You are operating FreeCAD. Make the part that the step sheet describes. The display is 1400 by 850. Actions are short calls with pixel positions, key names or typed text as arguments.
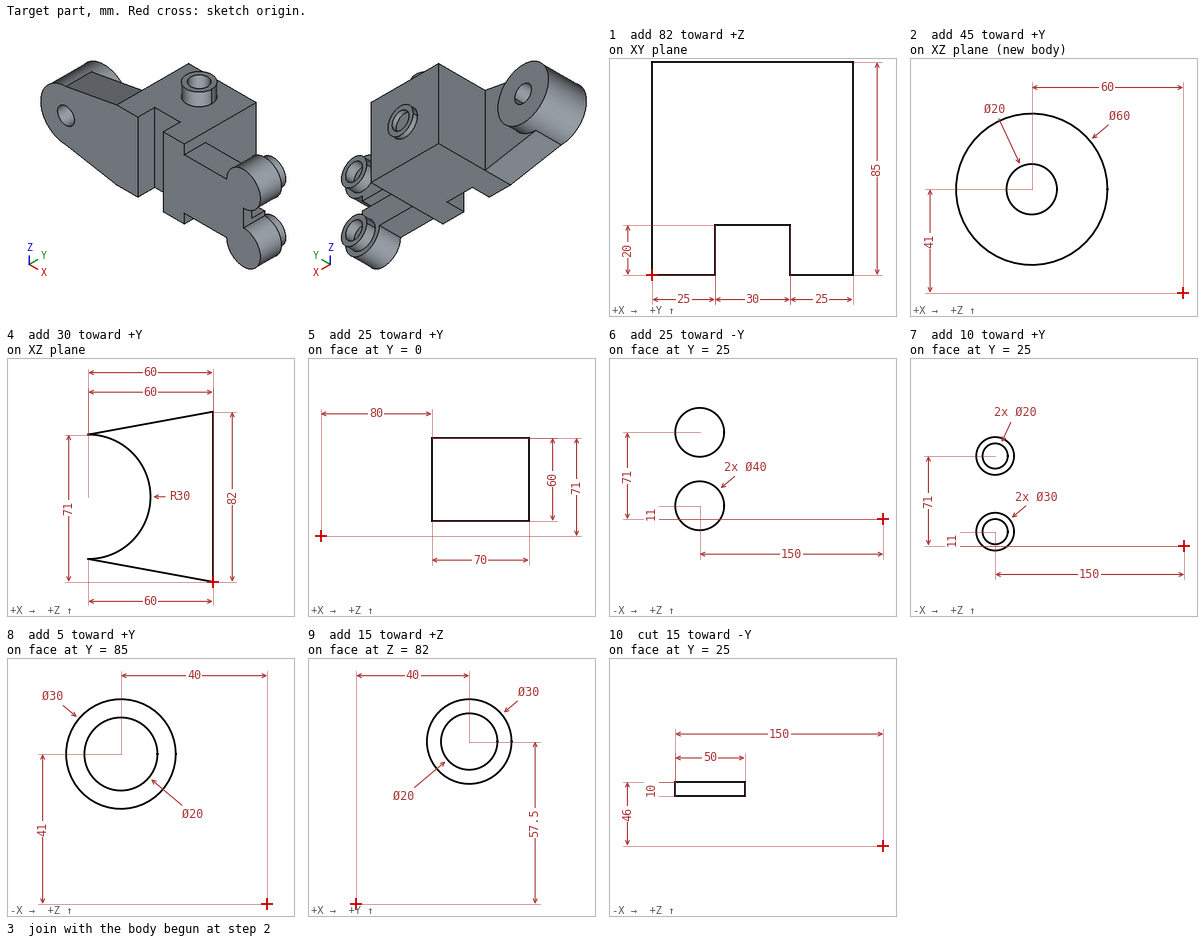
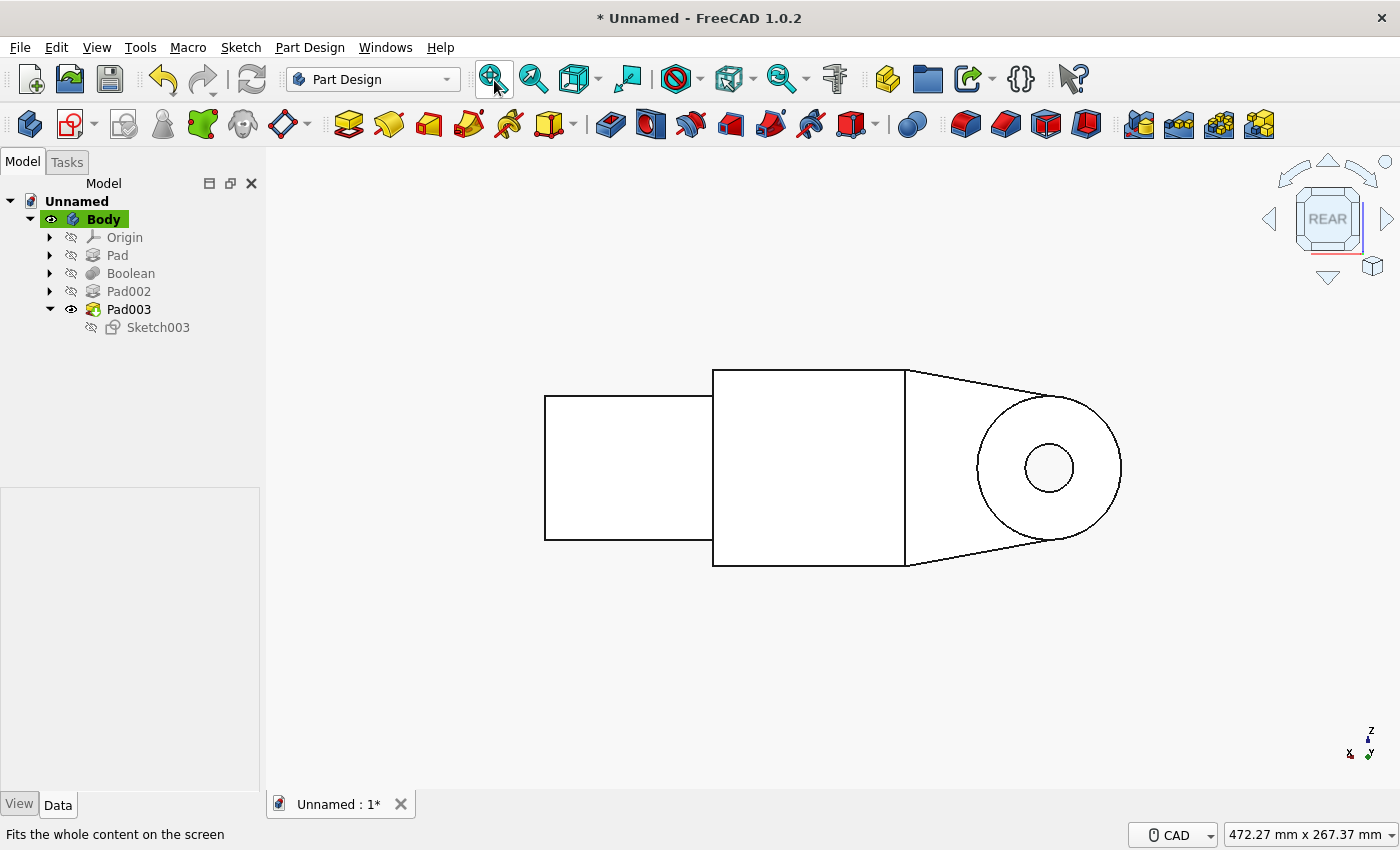
click(629, 467)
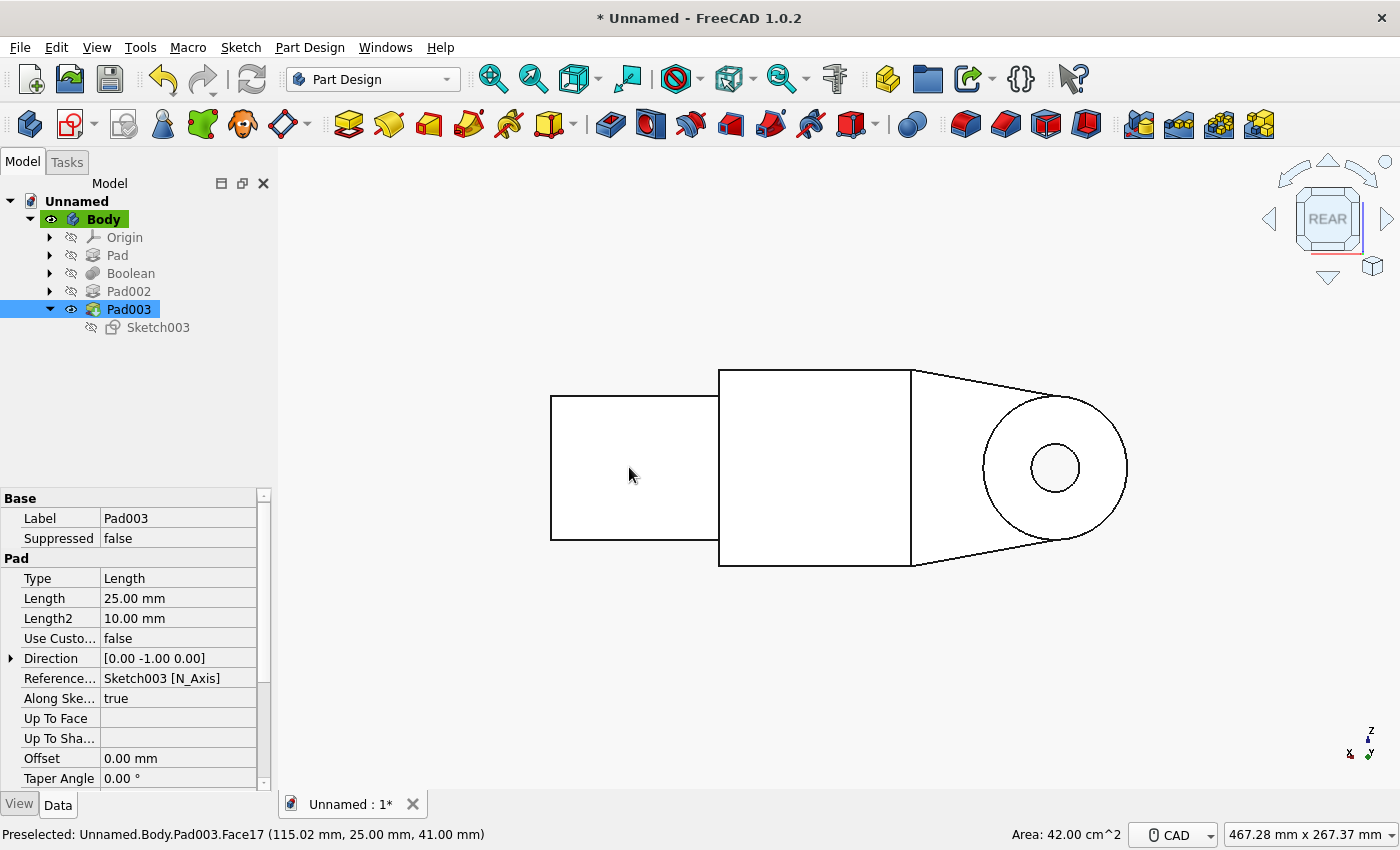
click(70, 124)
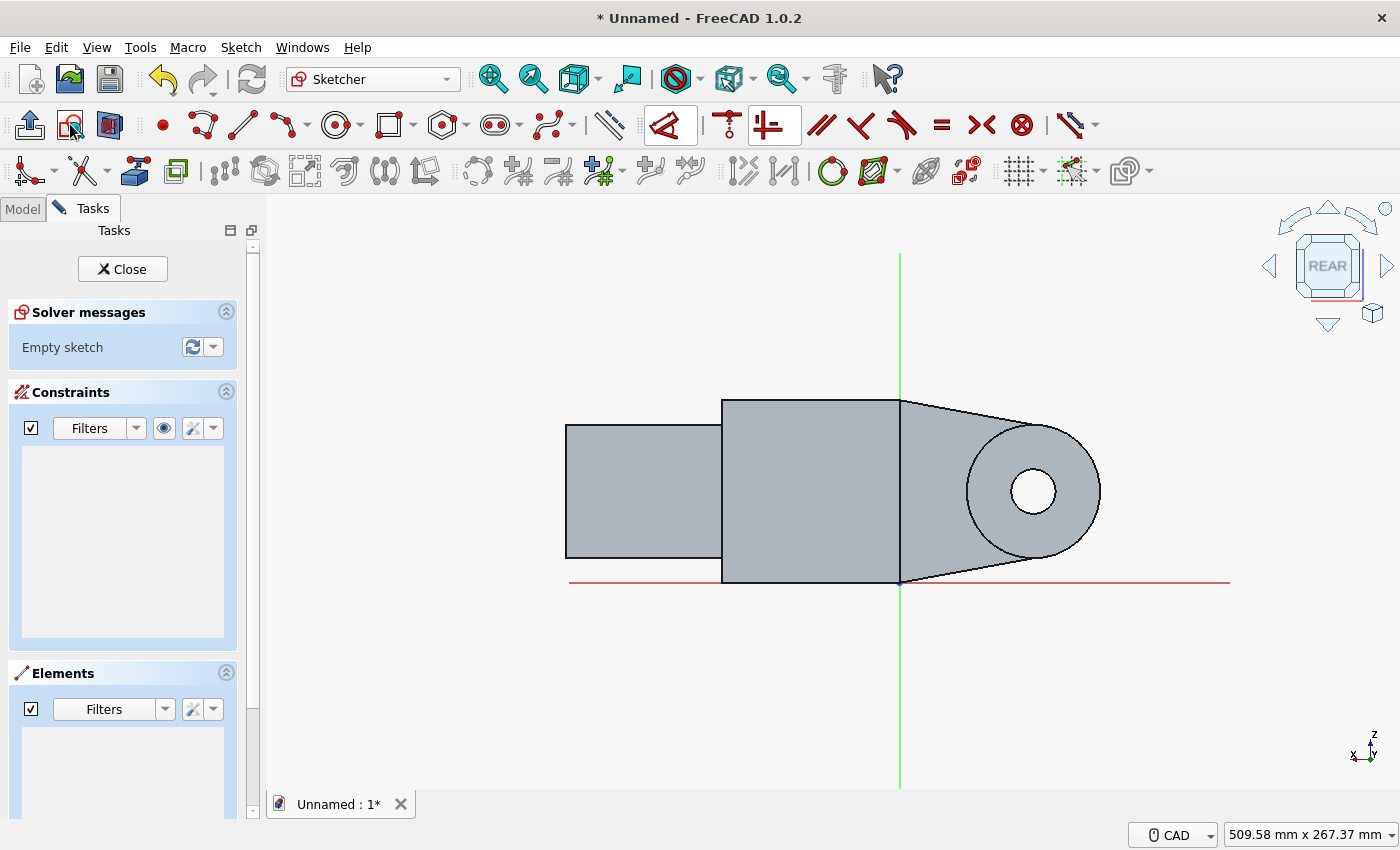
key(q)
key(s)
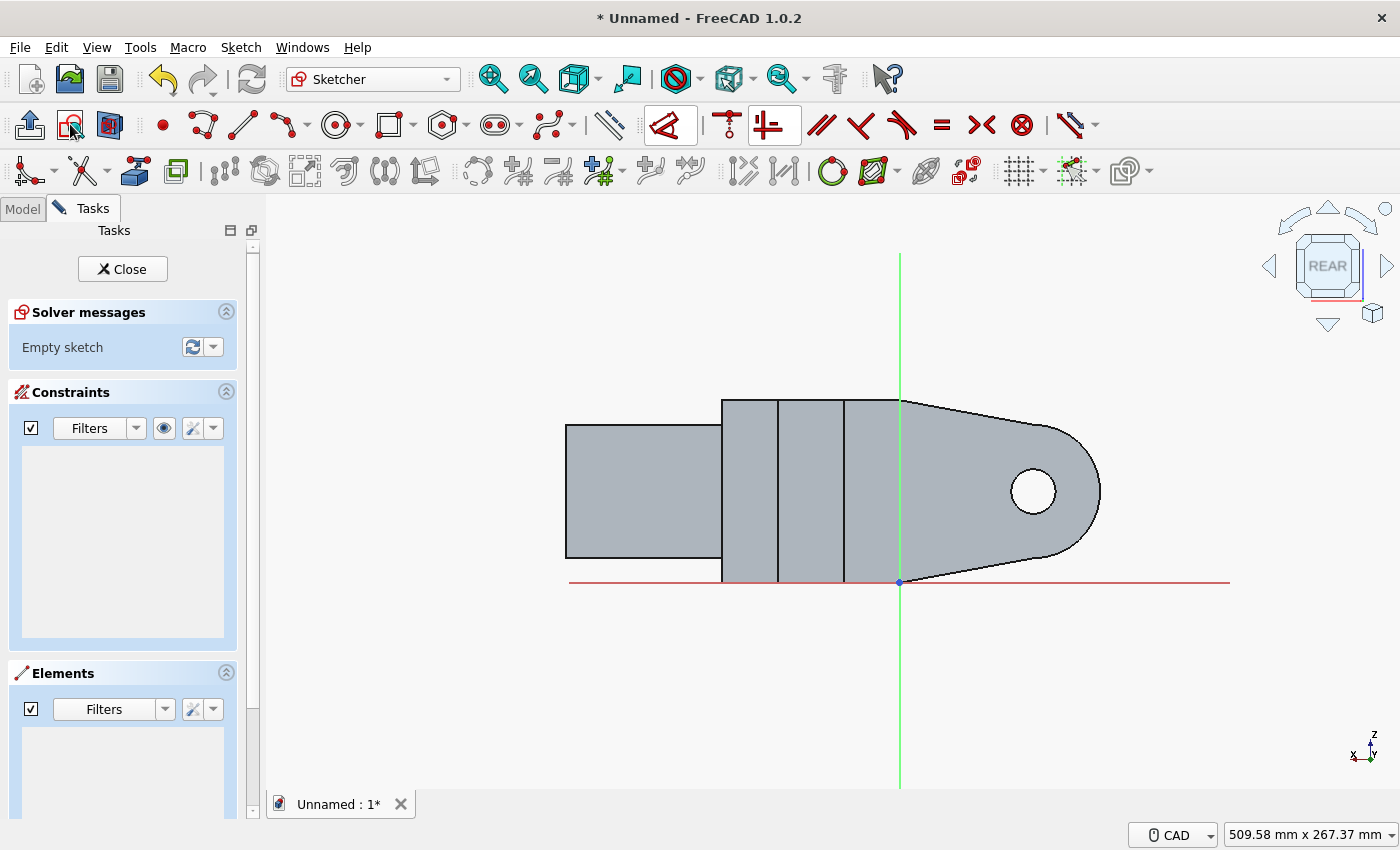
scroll(645, 491, up, 3)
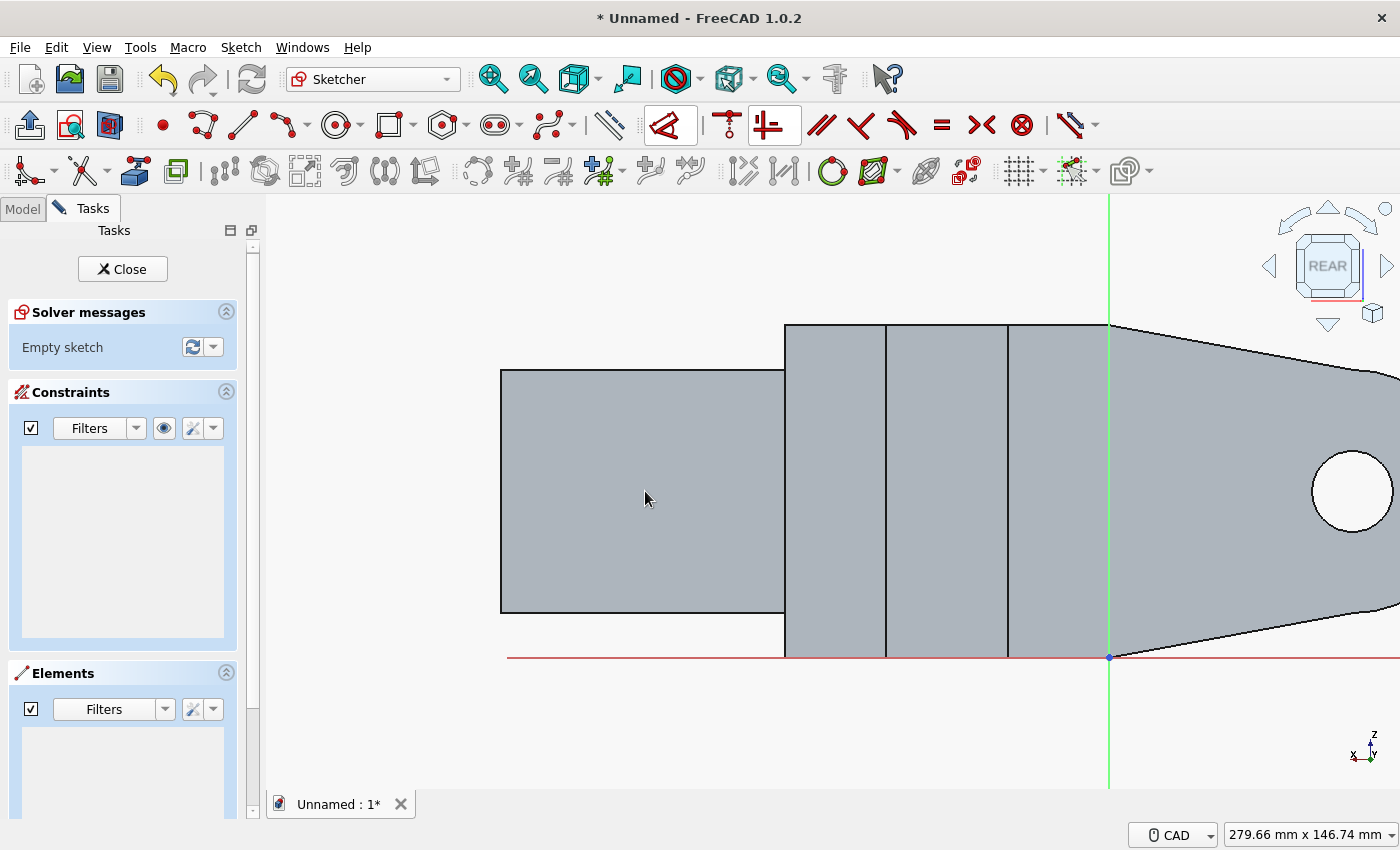
click(336, 126)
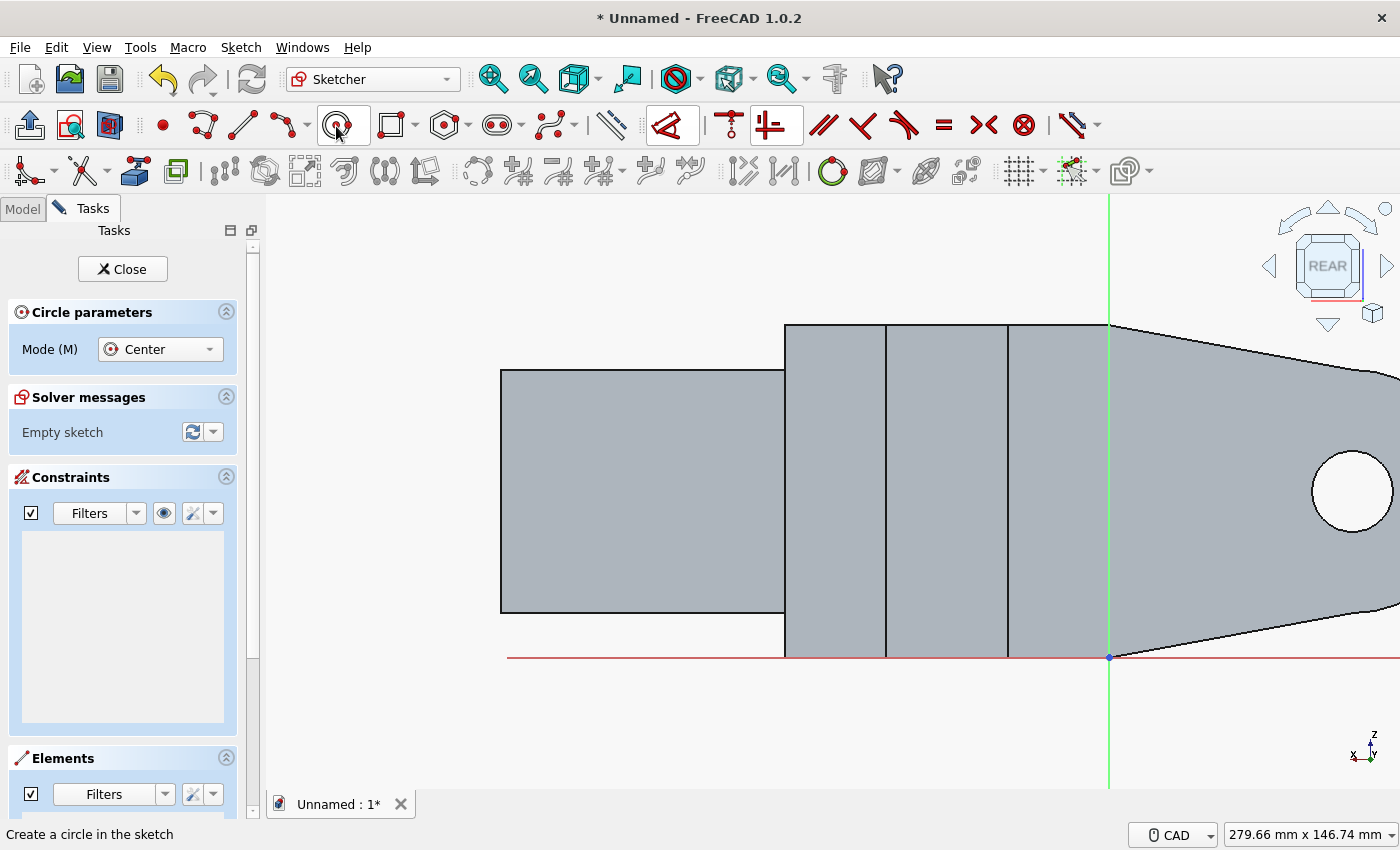
click(501, 613)
click(558, 556)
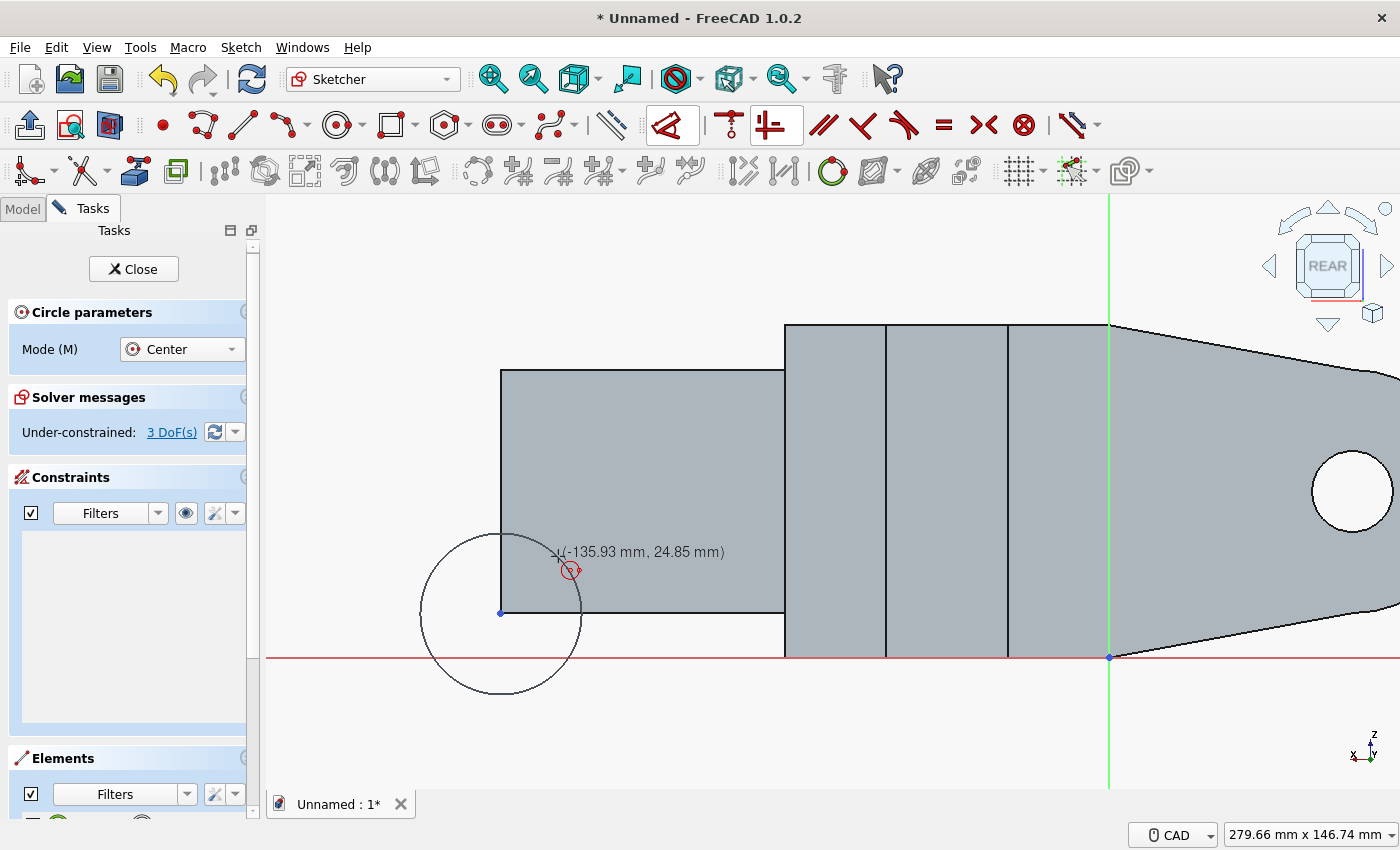
click(501, 370)
click(558, 313)
key(Escape)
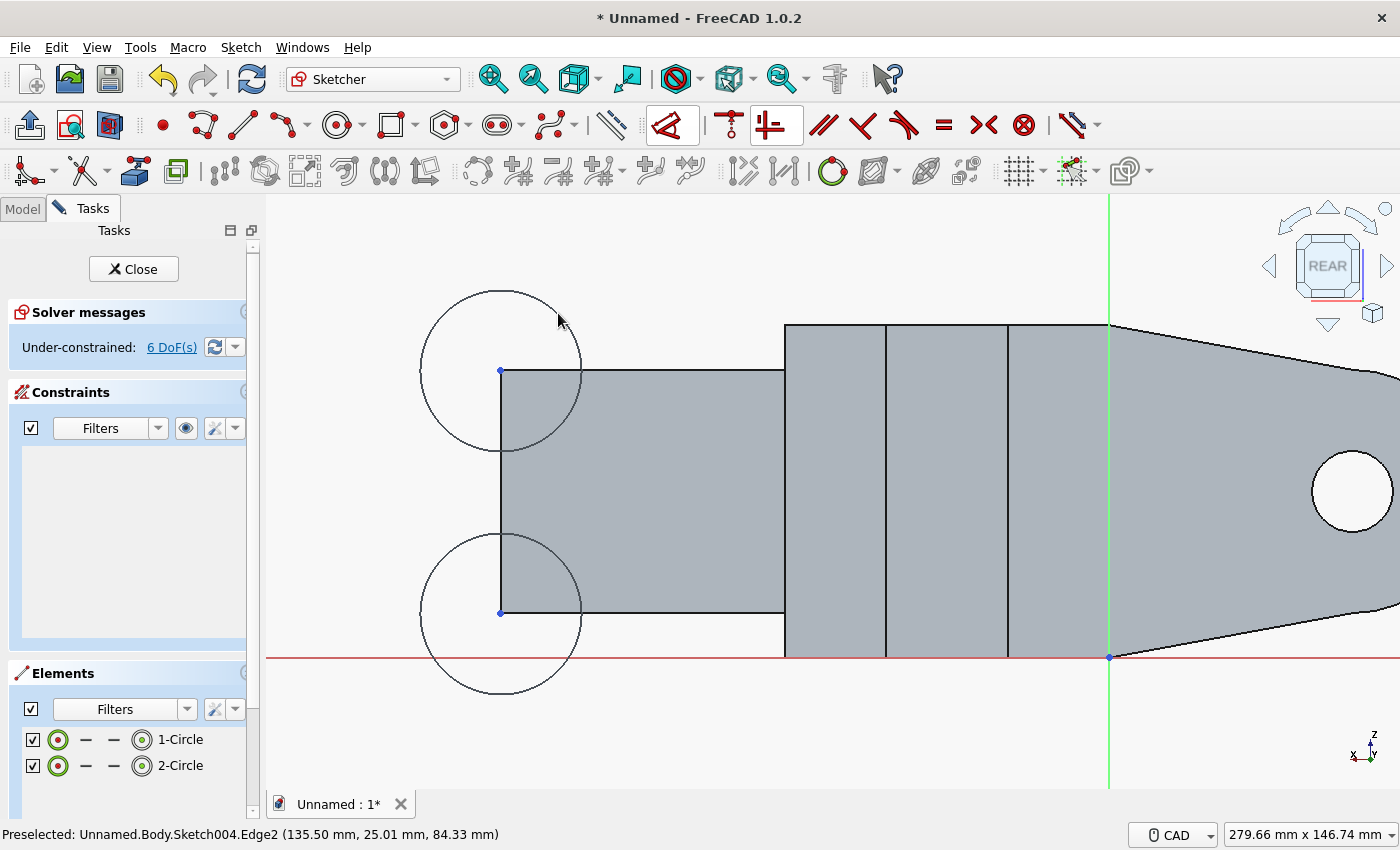
click(558, 557)